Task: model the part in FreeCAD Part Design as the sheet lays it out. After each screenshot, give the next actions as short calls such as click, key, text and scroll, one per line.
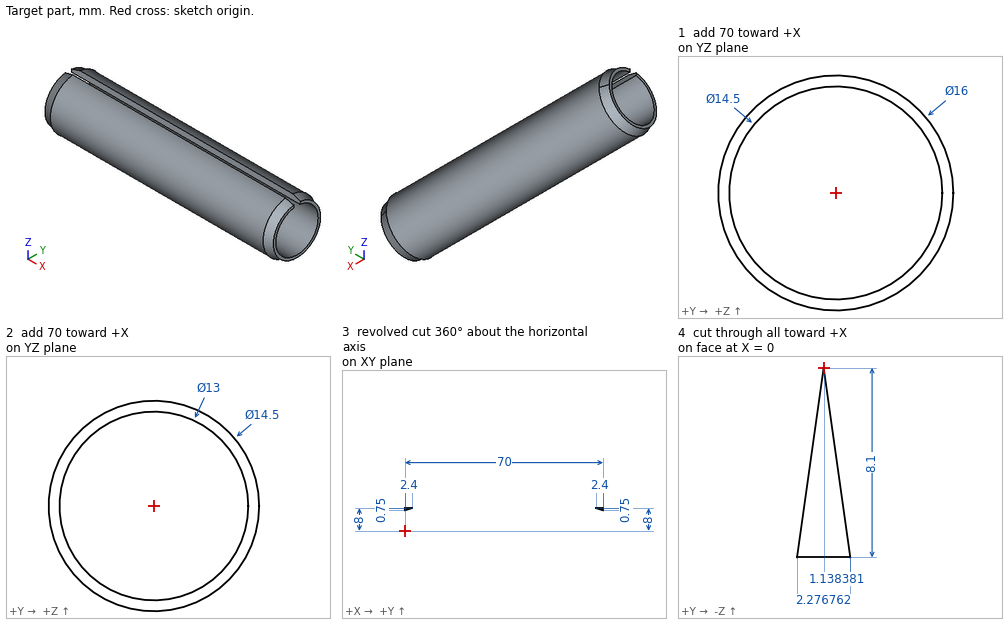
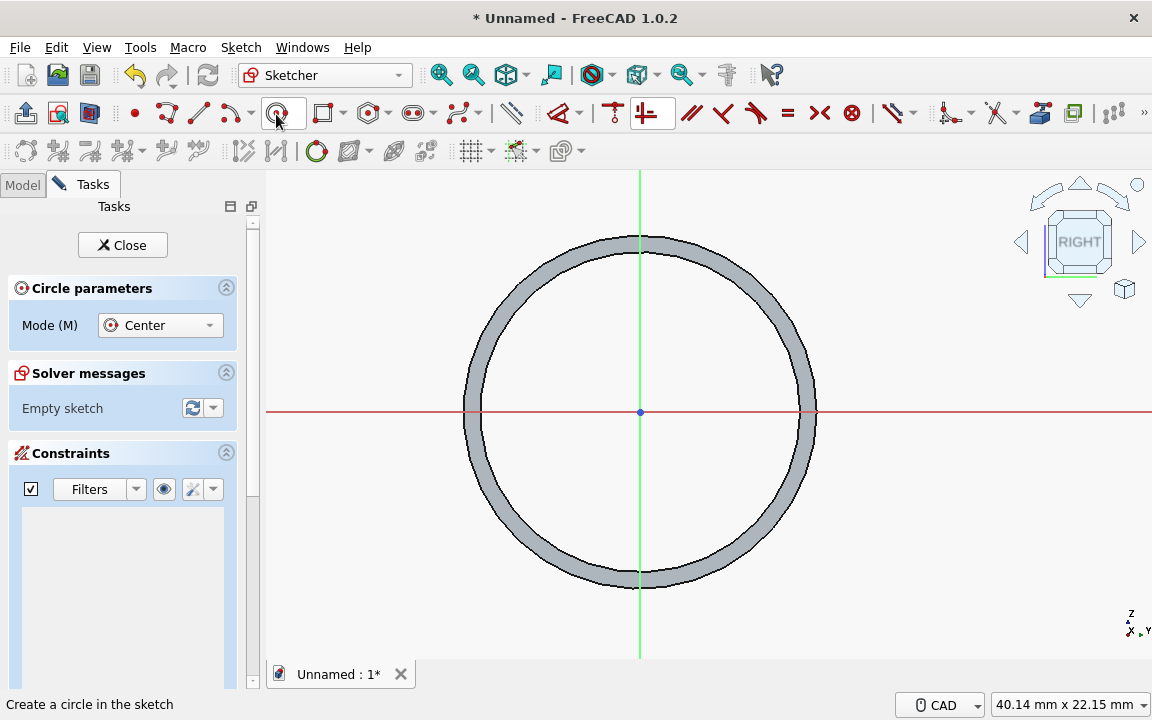
click(640, 412)
click(753, 299)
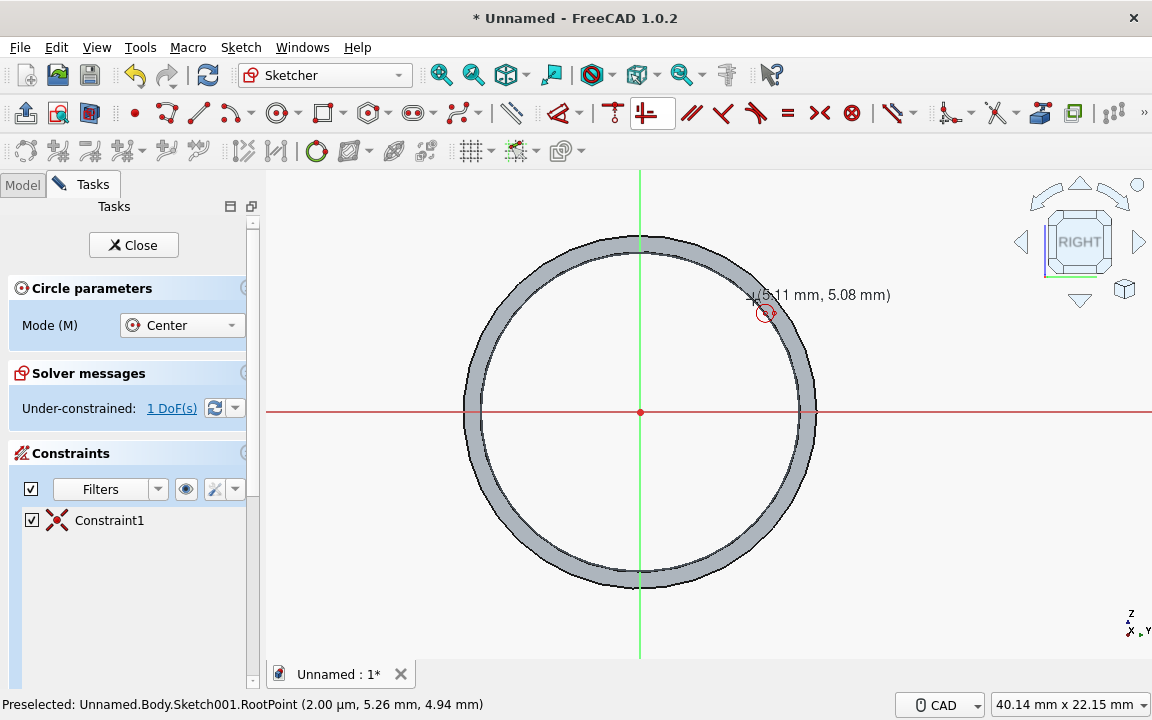
click(640, 412)
click(742, 311)
key(Escape)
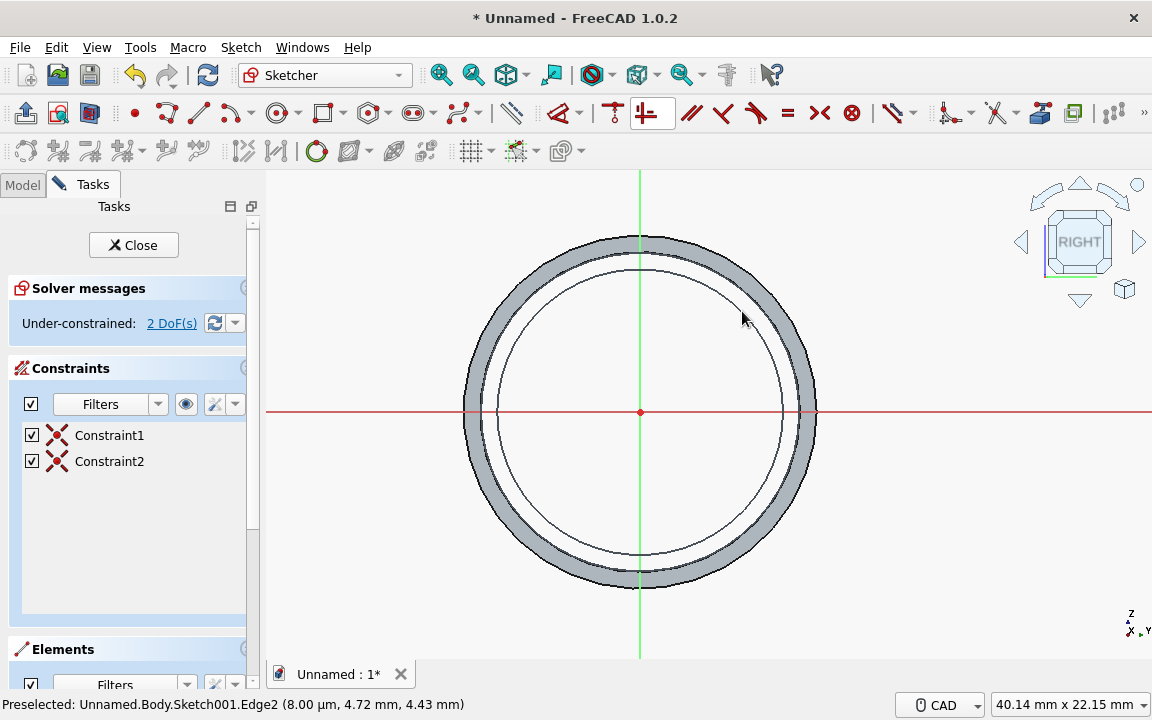
click(558, 114)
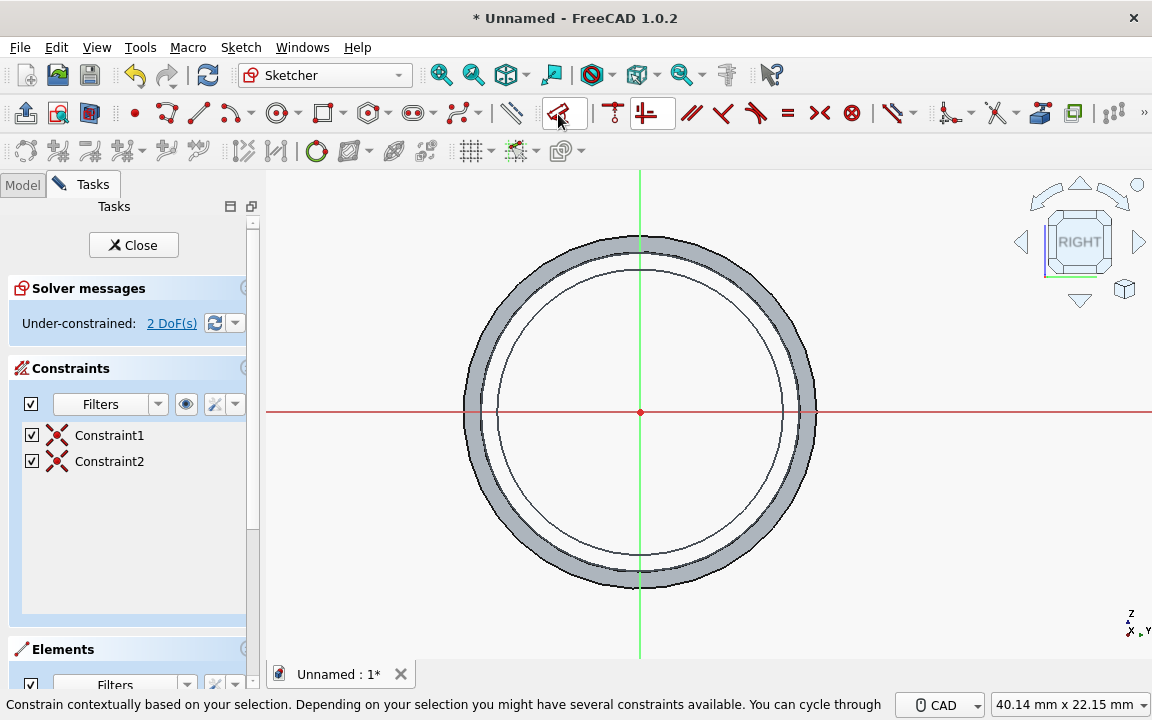
click(752, 299)
click(774, 276)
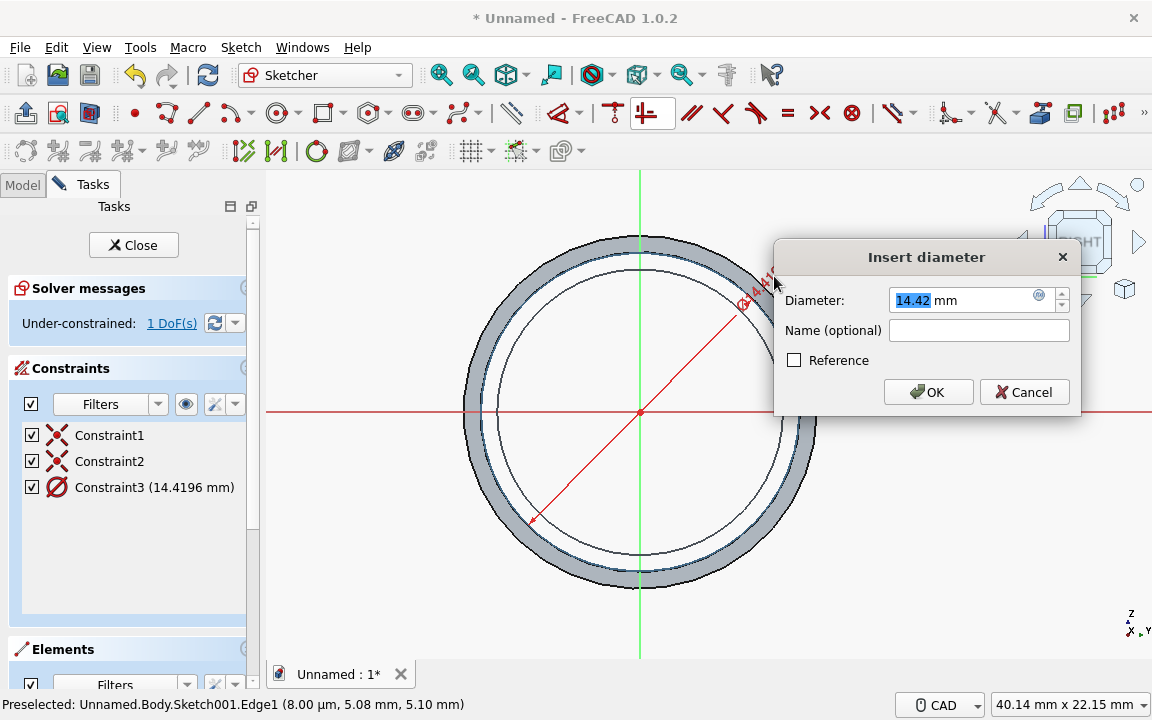
text(14.5)
key(Return)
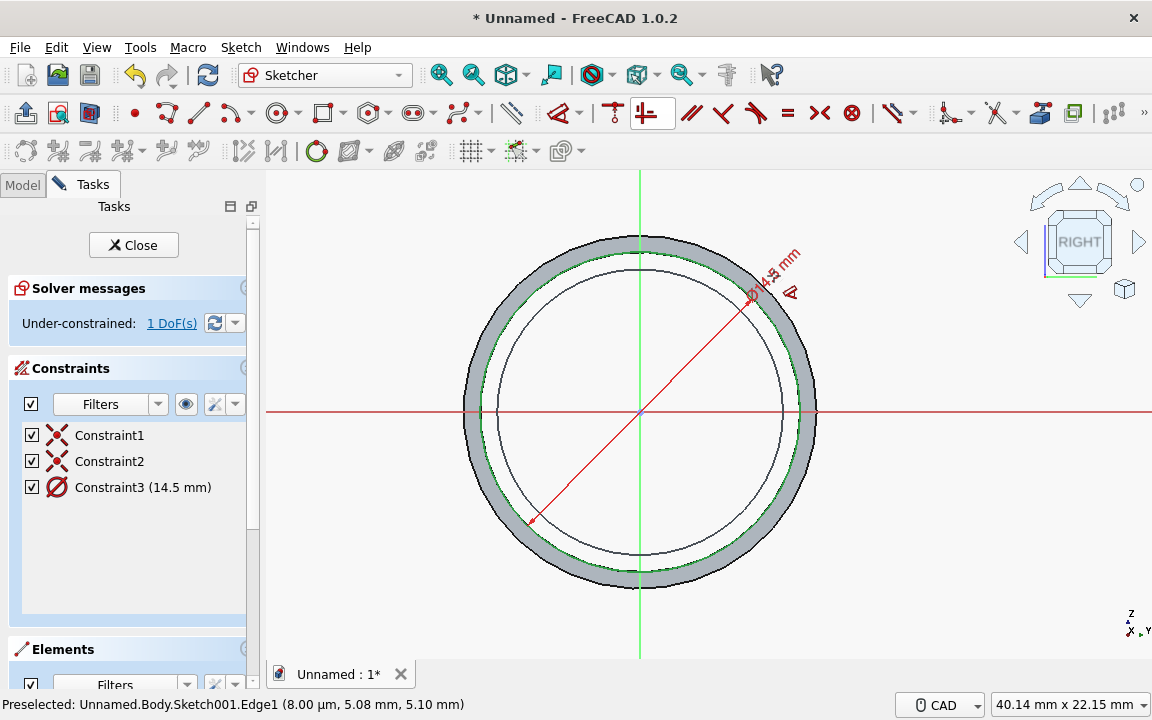
click(741, 311)
click(808, 363)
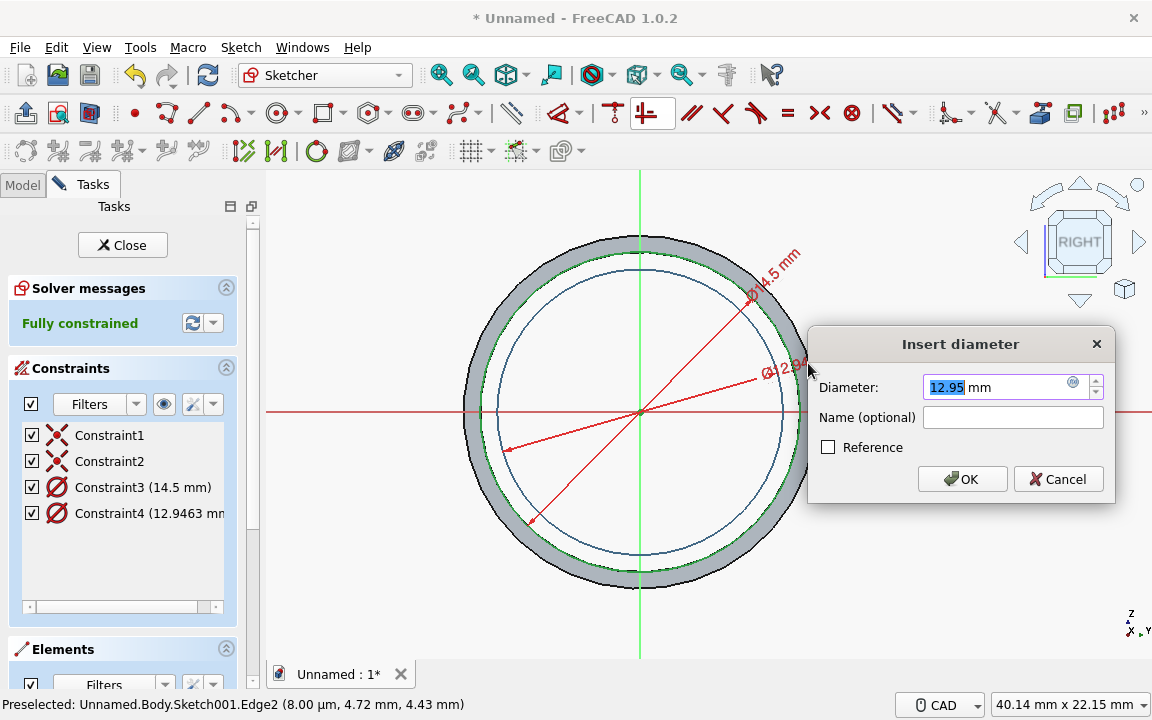
text(13)
key(Return)
key(Escape)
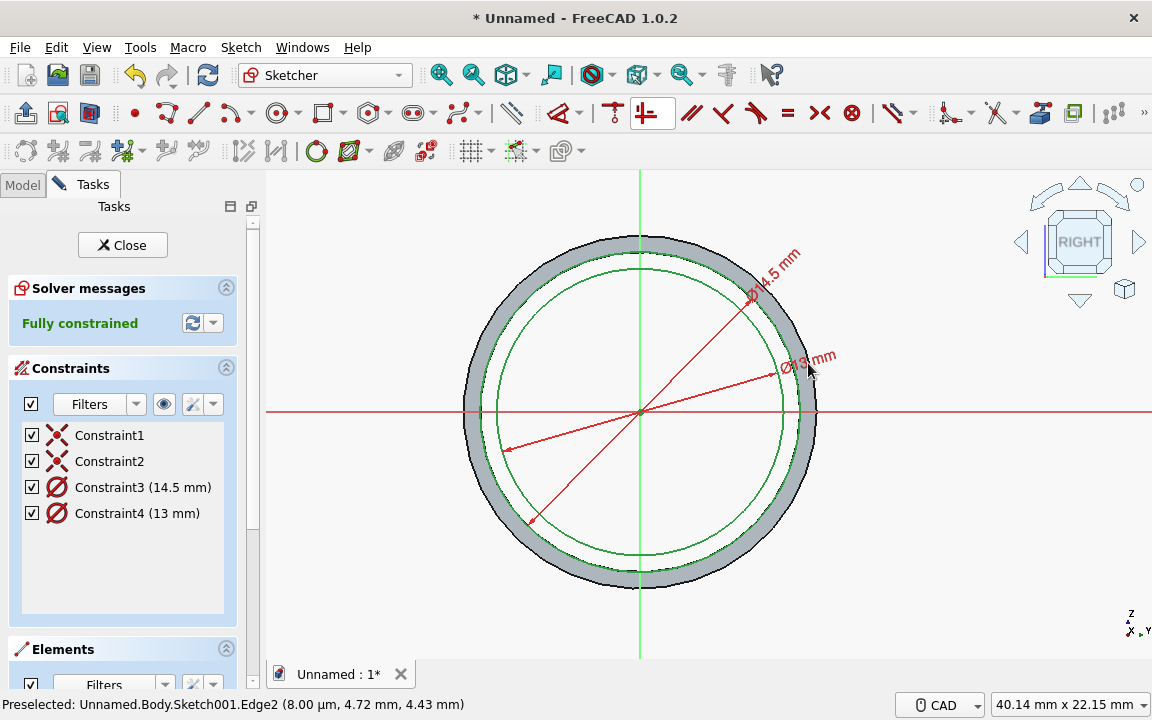
click(123, 245)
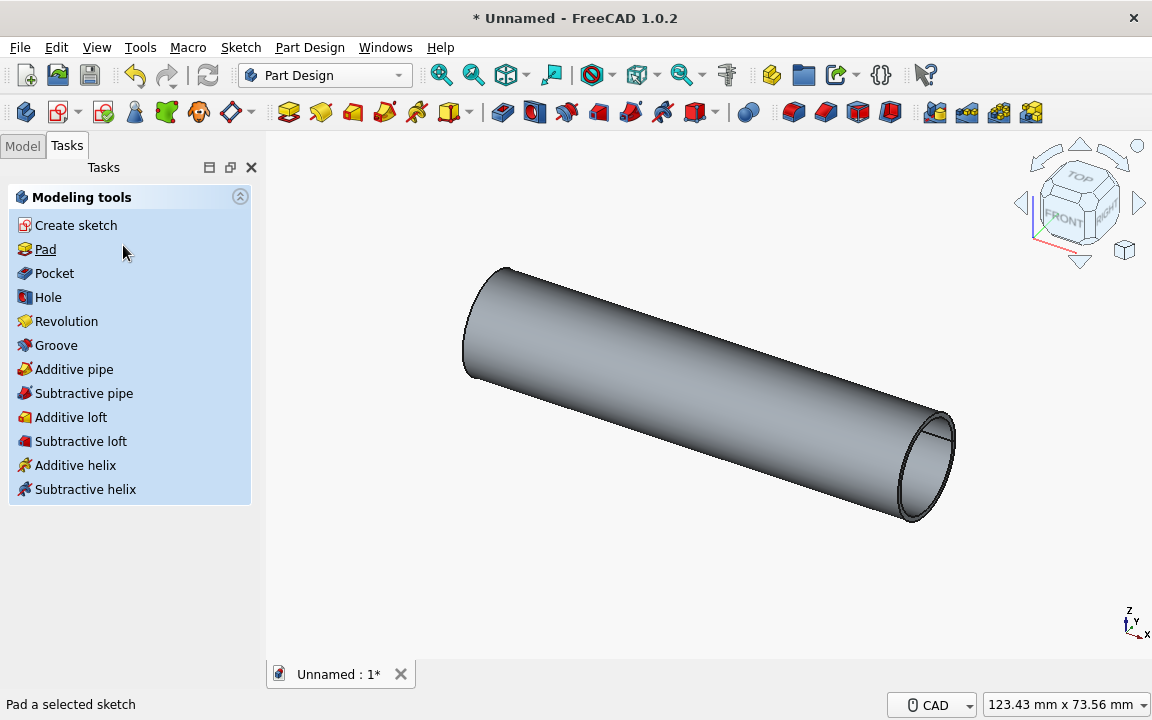
click(290, 112)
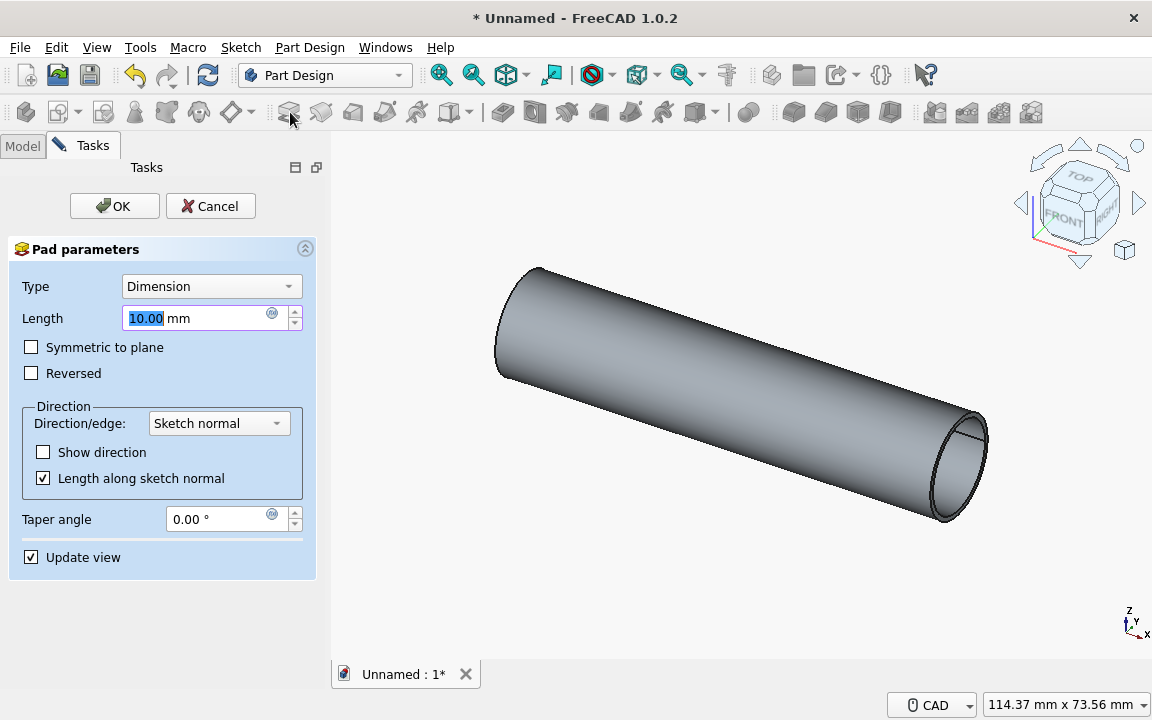
text(70)
key(Tab)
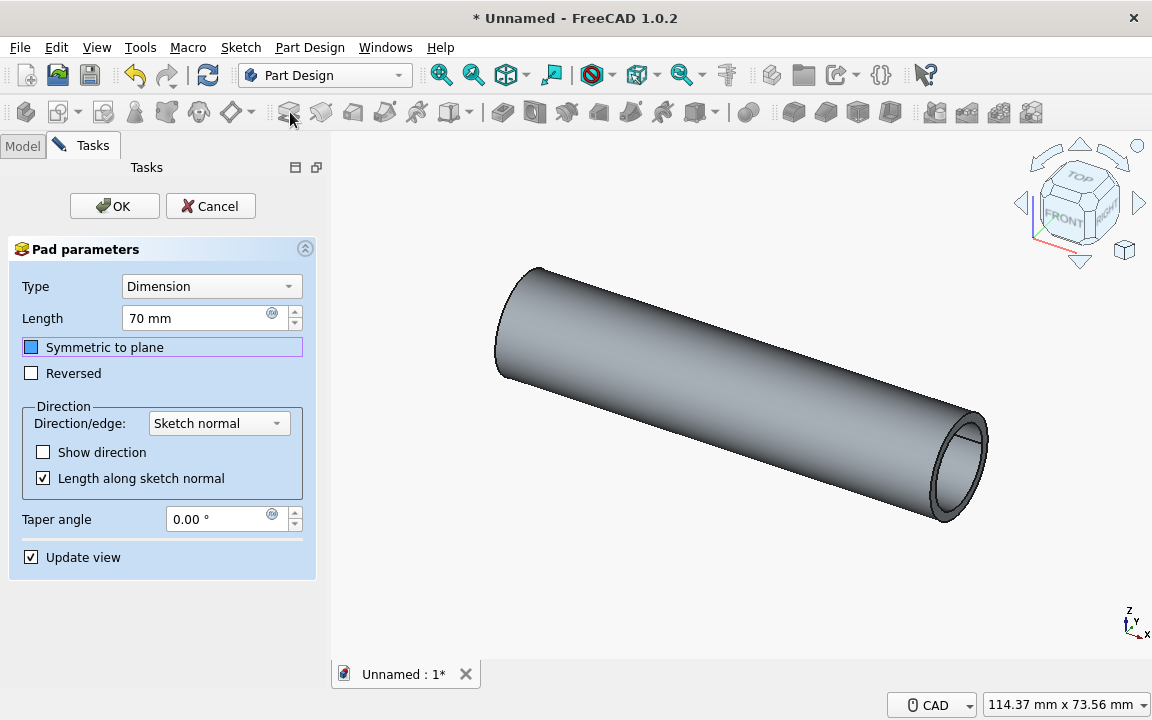
click(115, 206)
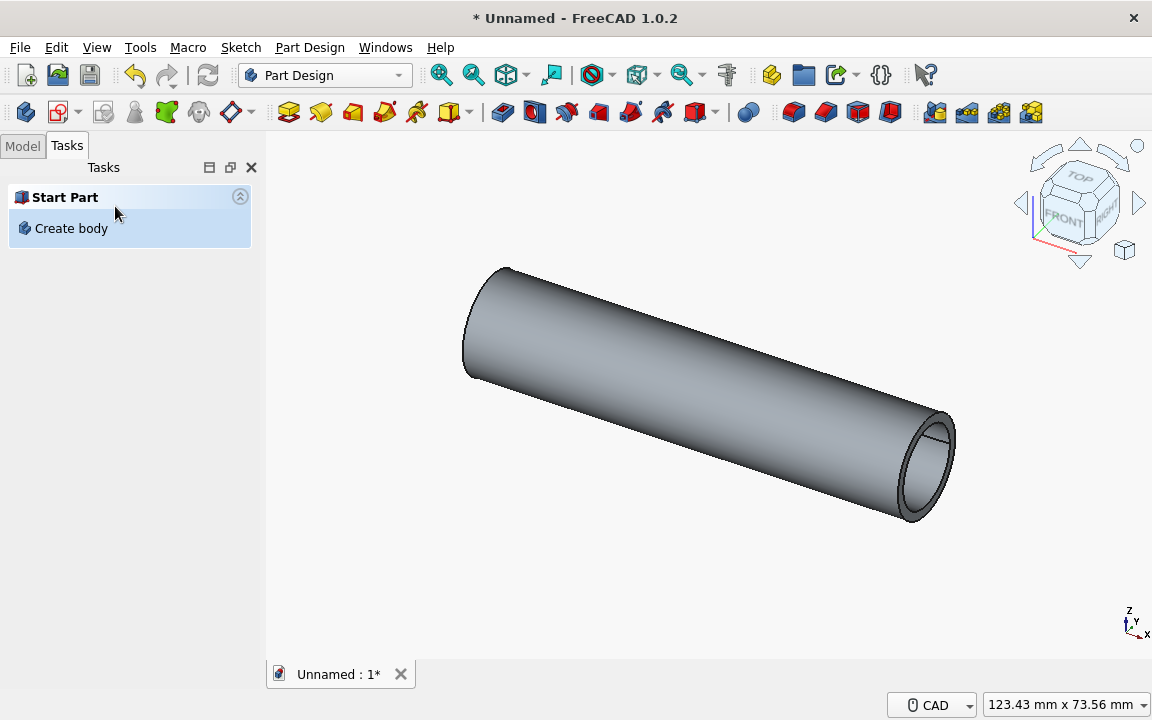
click(58, 112)